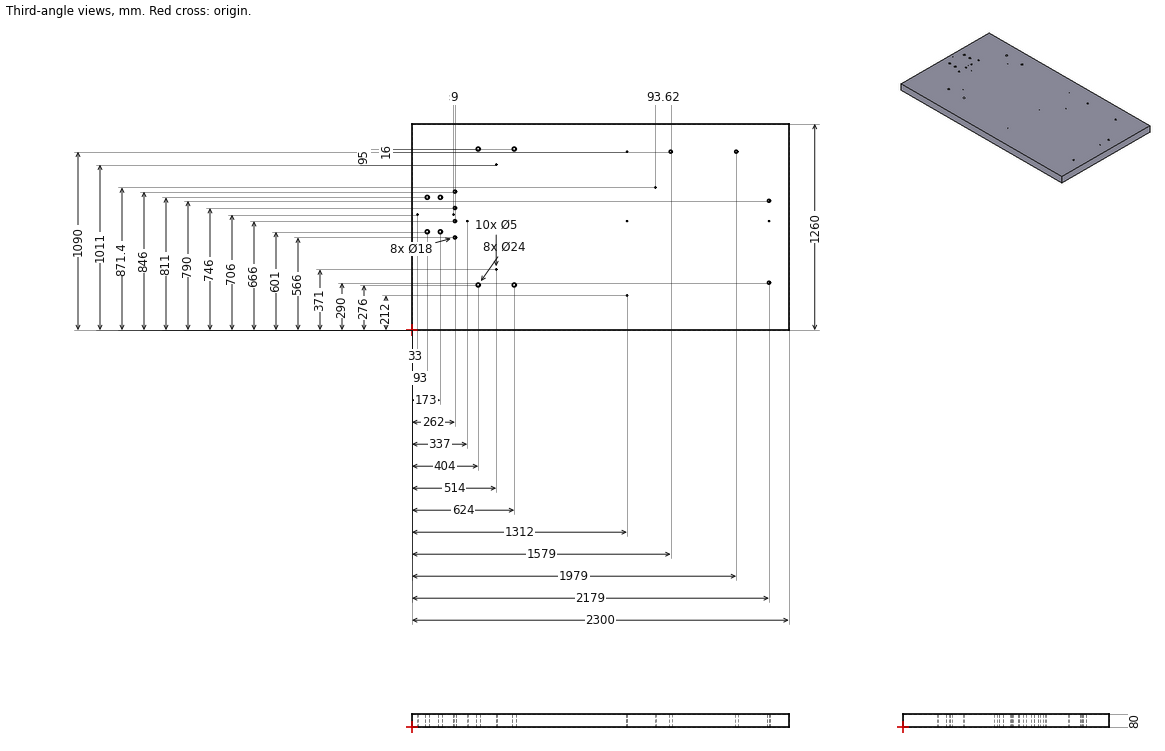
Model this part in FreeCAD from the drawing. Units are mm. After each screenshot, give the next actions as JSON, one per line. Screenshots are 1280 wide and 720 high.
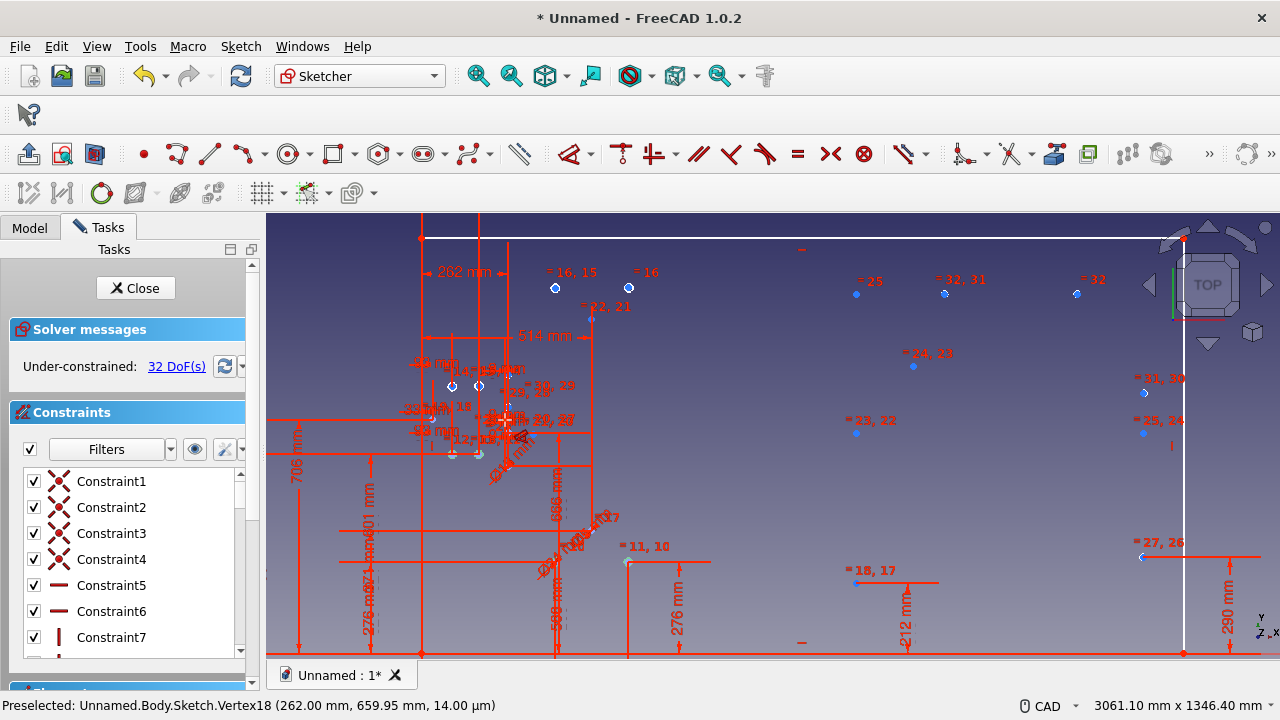
{"action": "left_click", "coordinate": [505, 420]}
{"action": "left_click", "coordinate": [388, 477]}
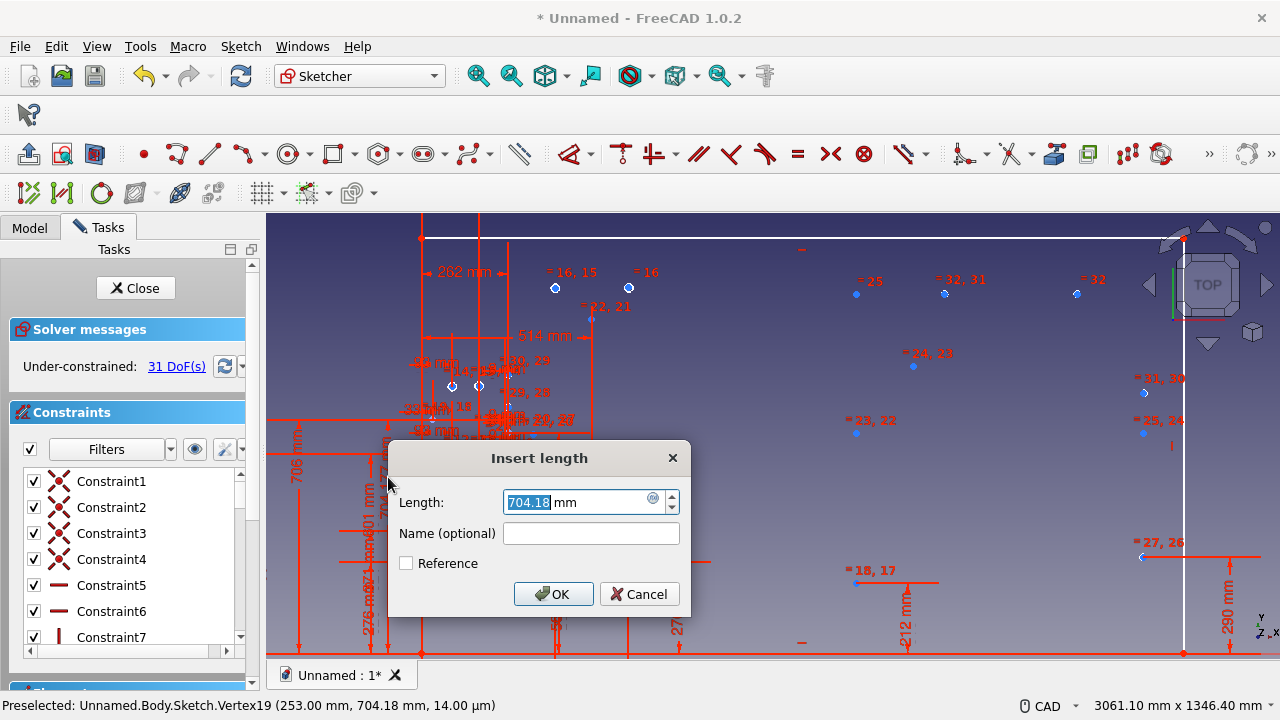
{"action": "type", "text": "706"}
{"action": "key", "text": "Return"}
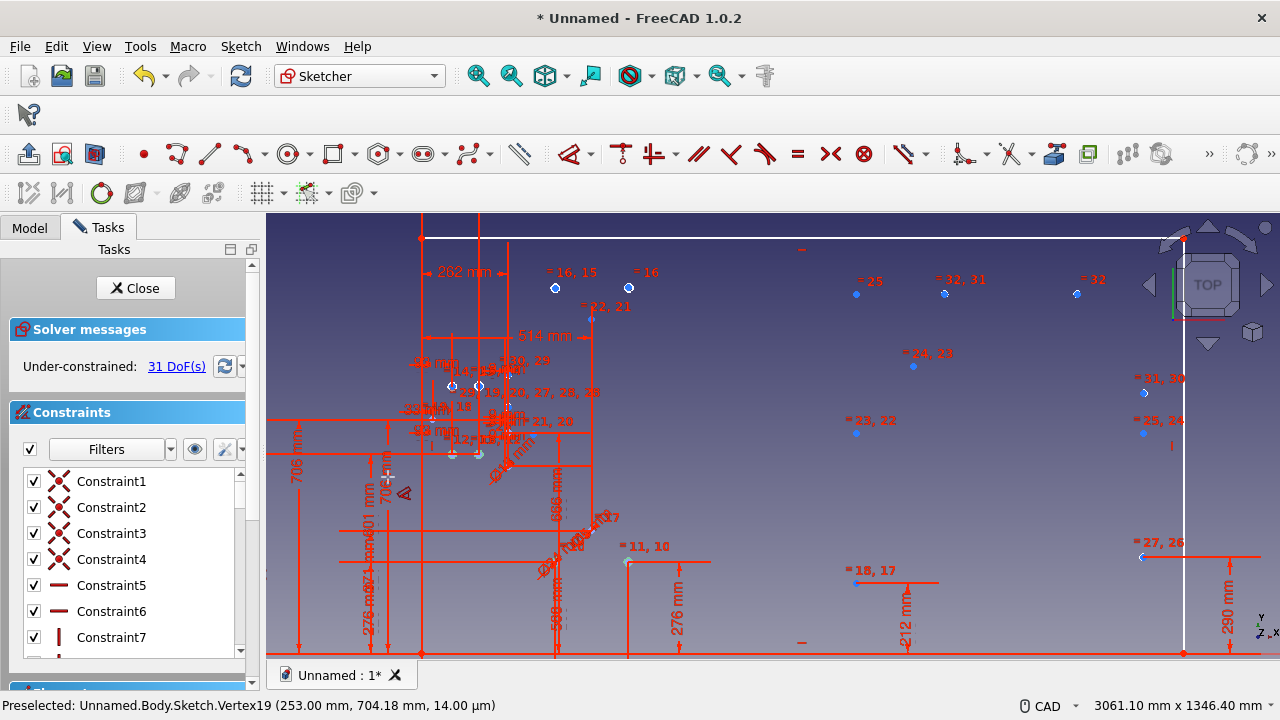
{"action": "left_click", "coordinate": [508, 407]}
{"action": "left_click", "coordinate": [590, 468]}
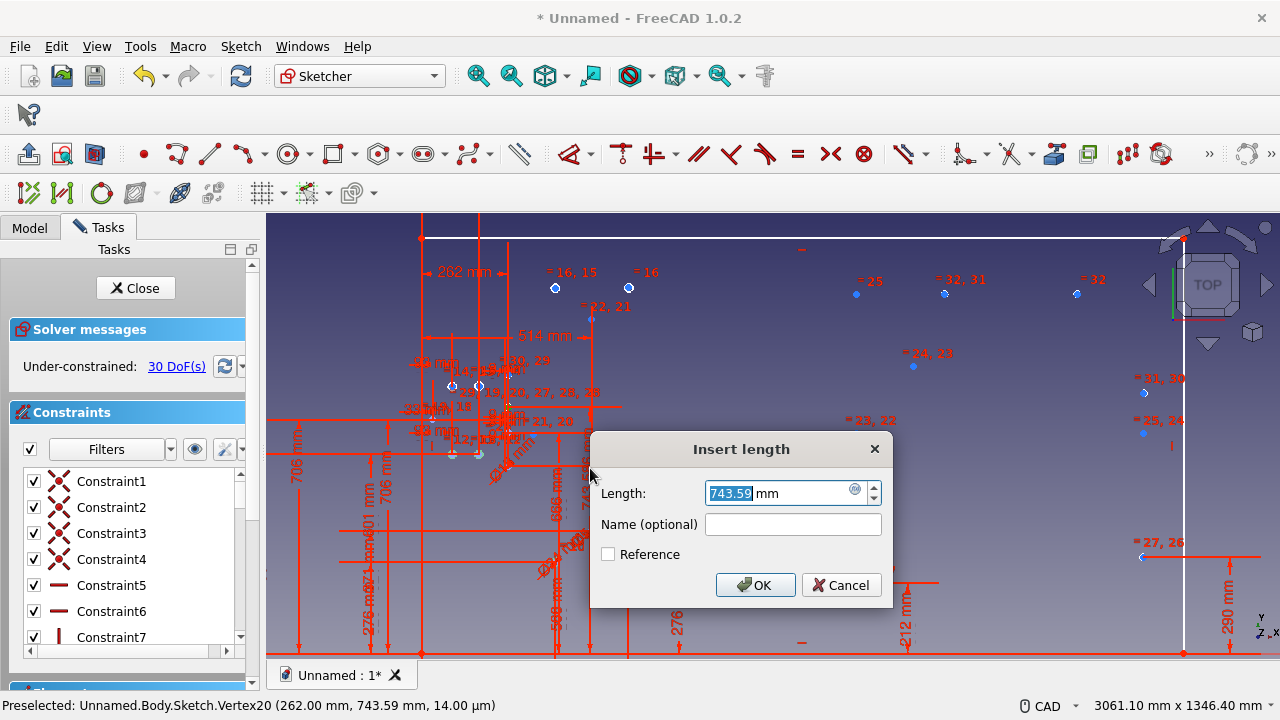
{"action": "type", "text": "746"}
{"action": "key", "text": "Return"}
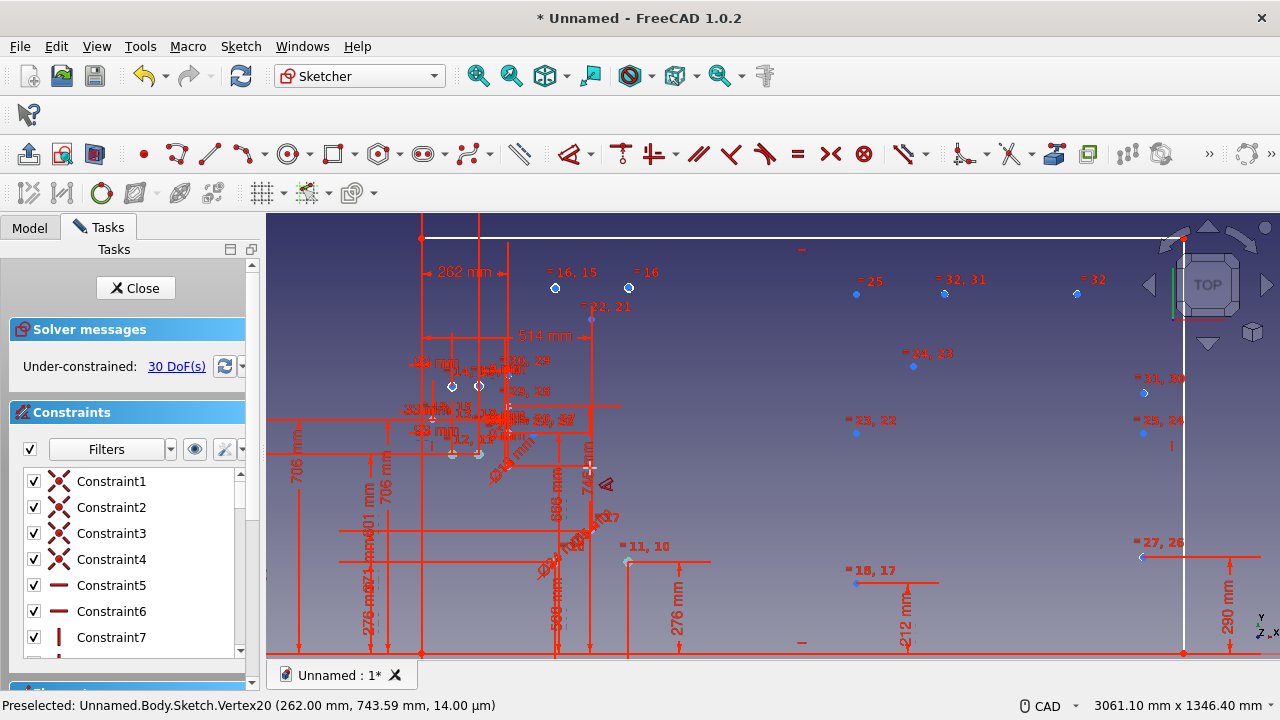
{"action": "left_click", "coordinate": [533, 434]}
{"action": "left_click", "coordinate": [452, 328]}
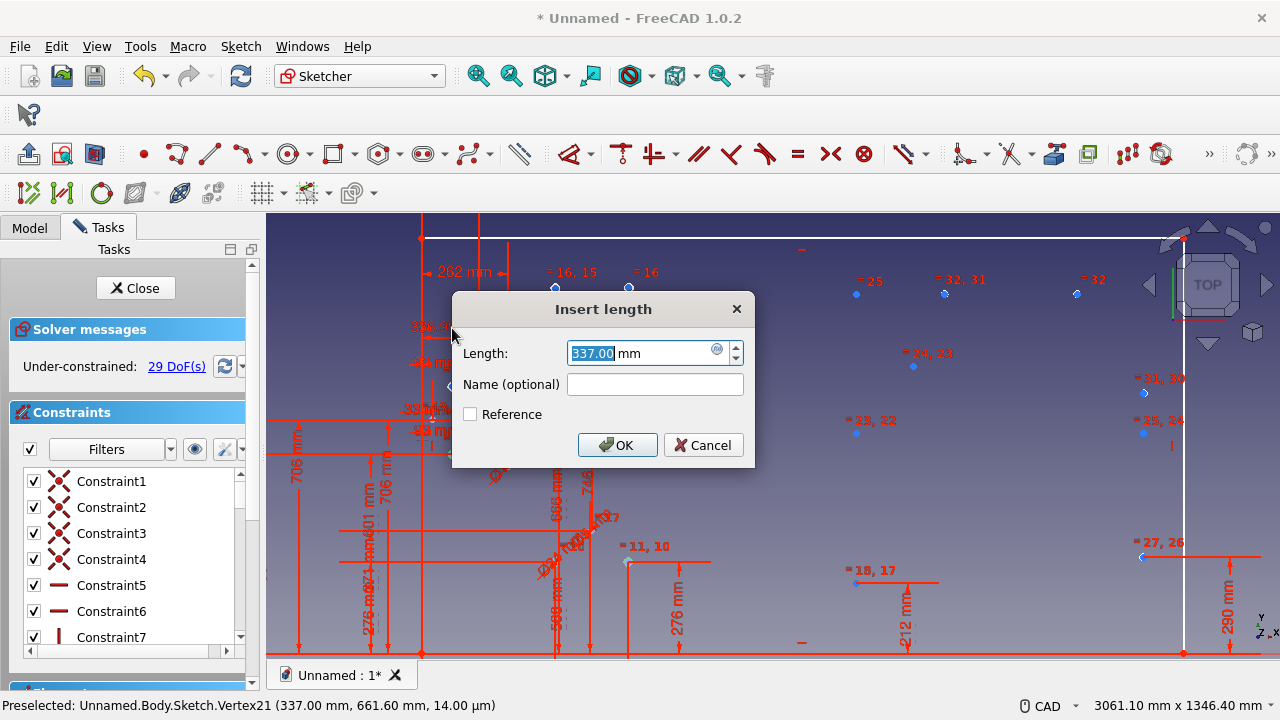
{"action": "type", "text": "337"}
{"action": "key", "text": "Return"}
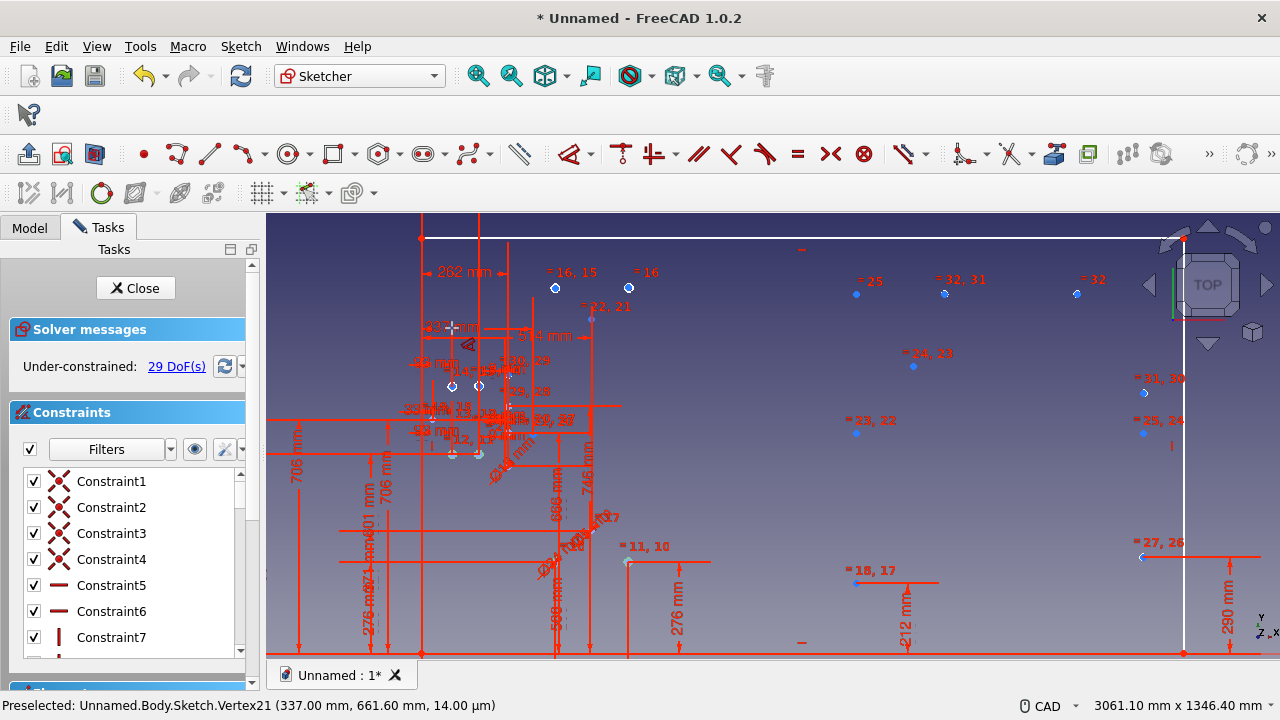
{"action": "left_click", "coordinate": [533, 434]}
{"action": "left_click", "coordinate": [388, 533]}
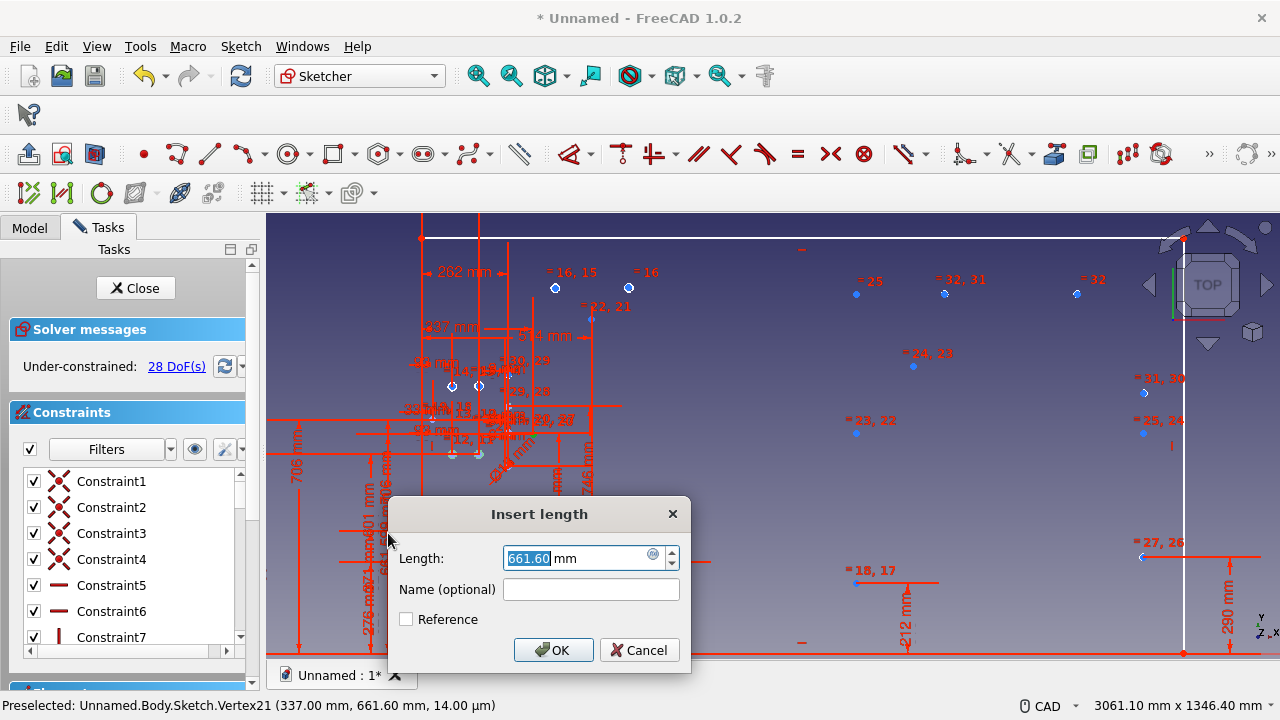
{"action": "type", "text": "666"}
{"action": "key", "text": "Return"}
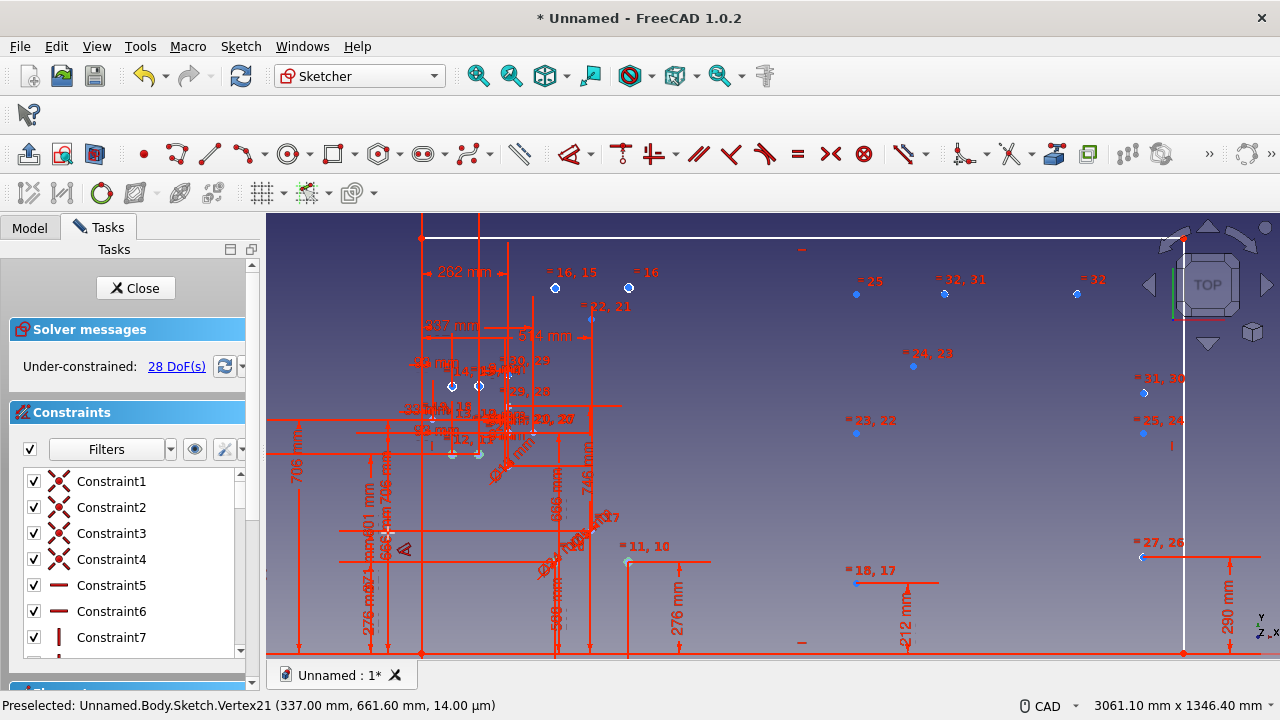
{"action": "left_click", "coordinate": [452, 387]}
{"action": "left_click", "coordinate": [486, 509]}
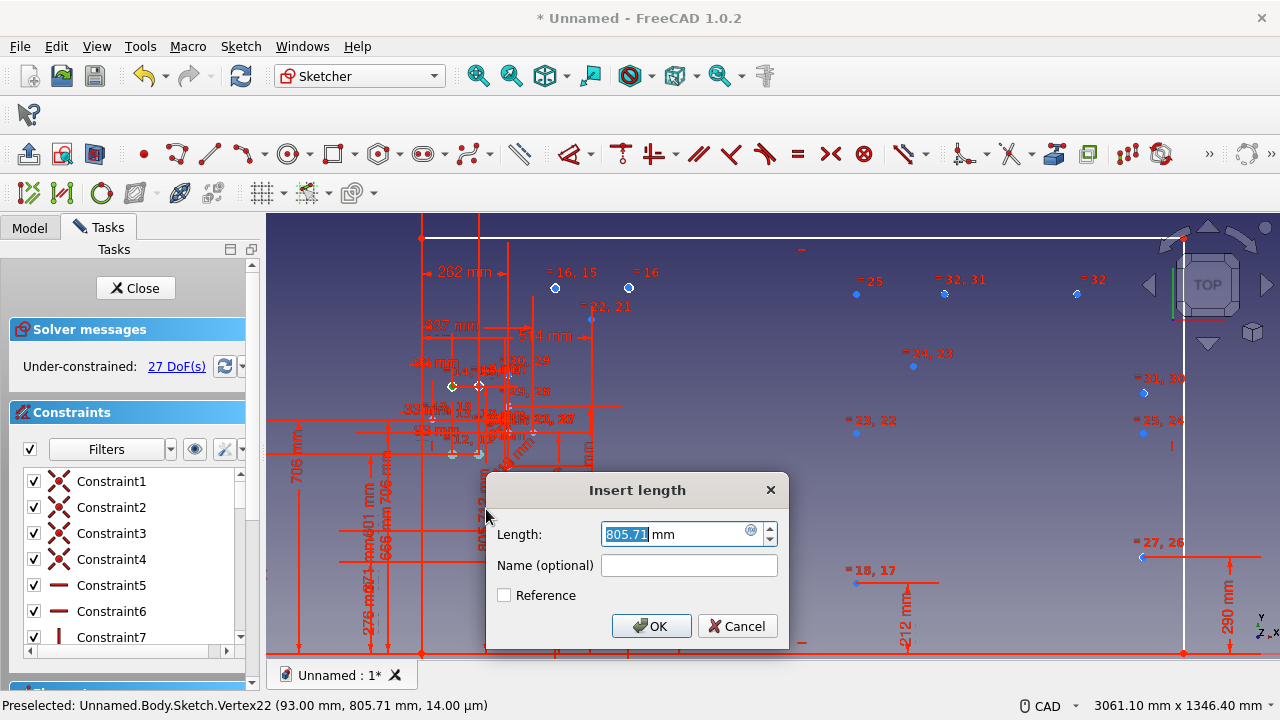
{"action": "type", "text": "811"}
{"action": "key", "text": "Return"}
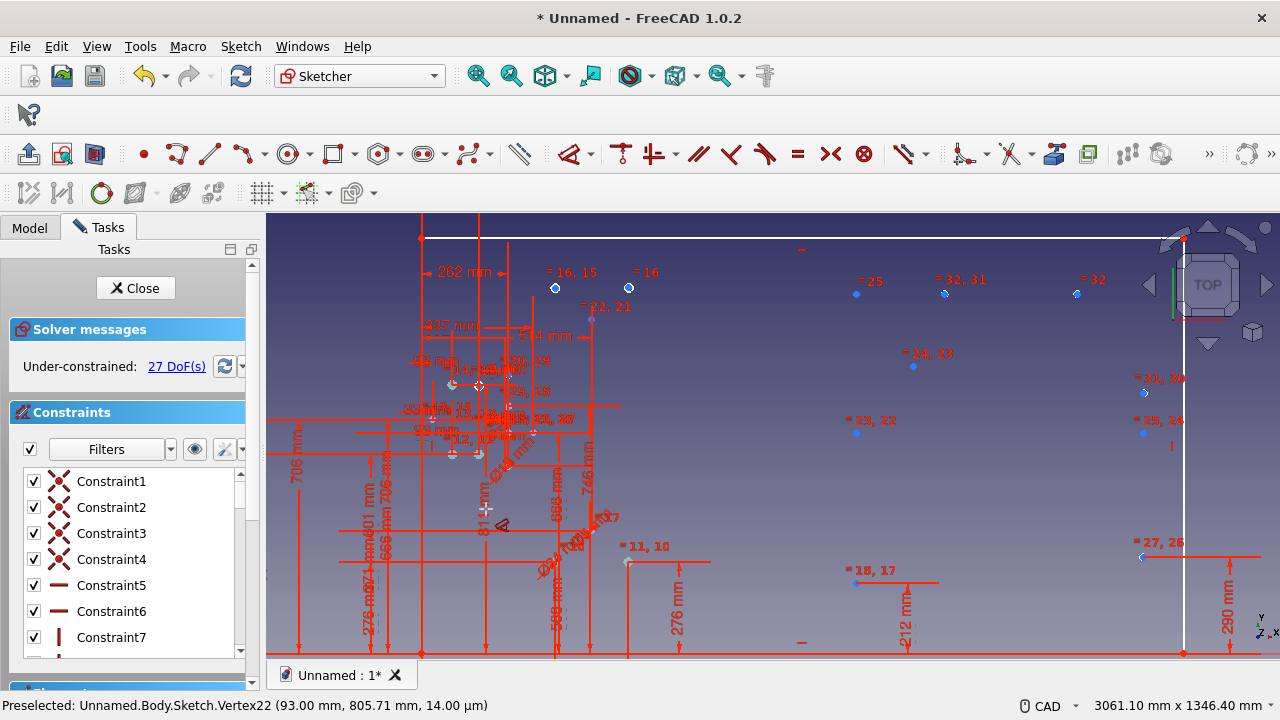
{"action": "left_click", "coordinate": [479, 386]}
{"action": "left_click", "coordinate": [450, 304]}